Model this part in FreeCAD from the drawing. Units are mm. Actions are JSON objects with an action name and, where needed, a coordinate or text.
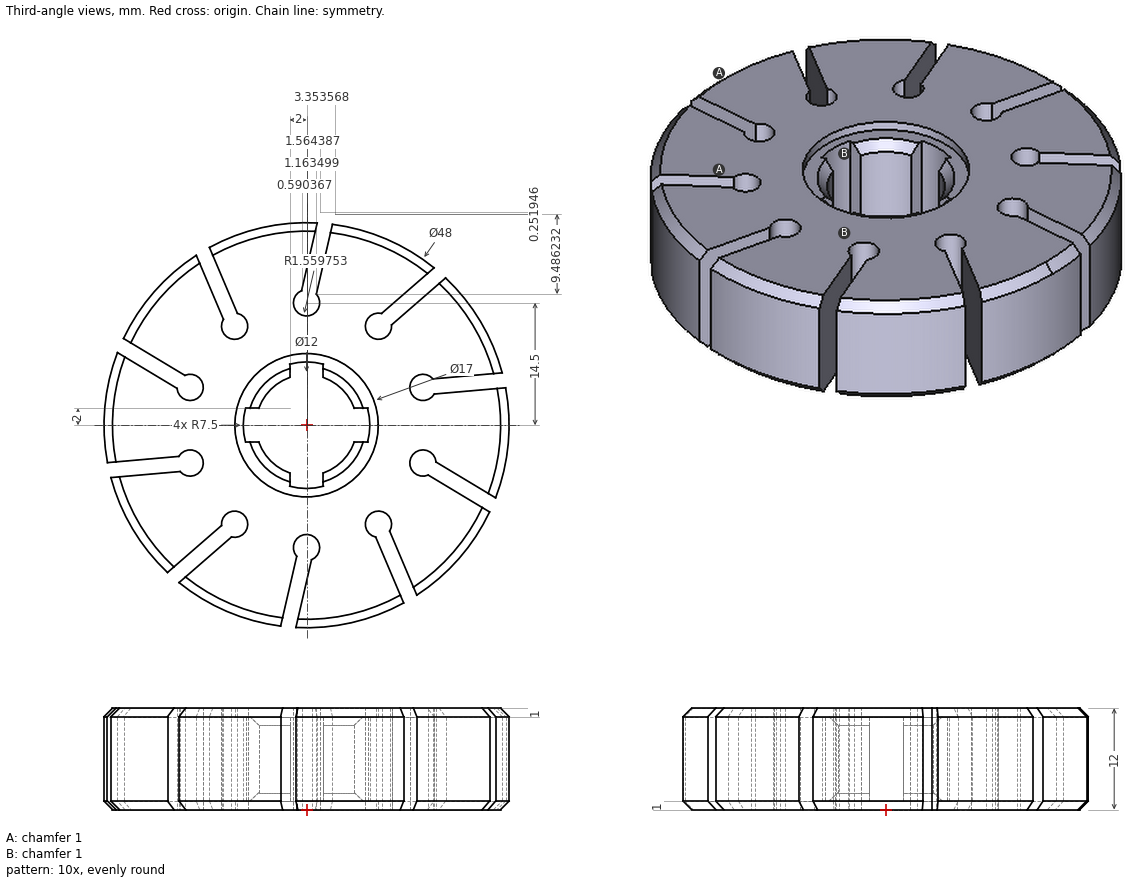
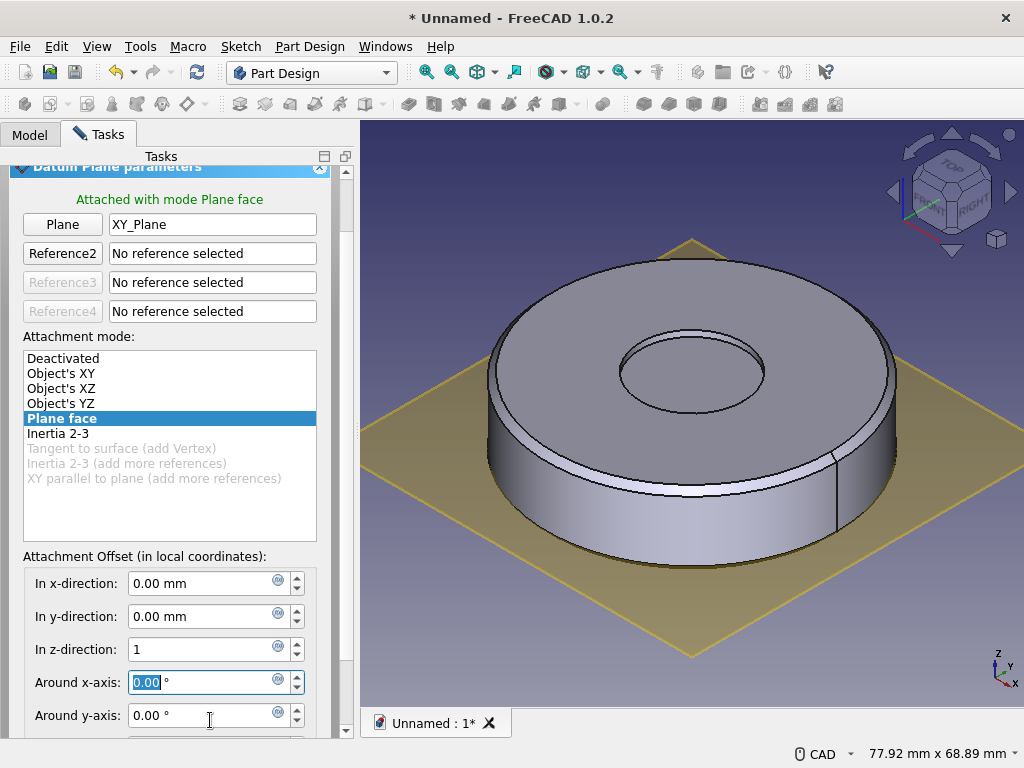
{"action": "scroll", "coordinate": [346, 452], "scroll_direction": "up", "scroll_amount": 2}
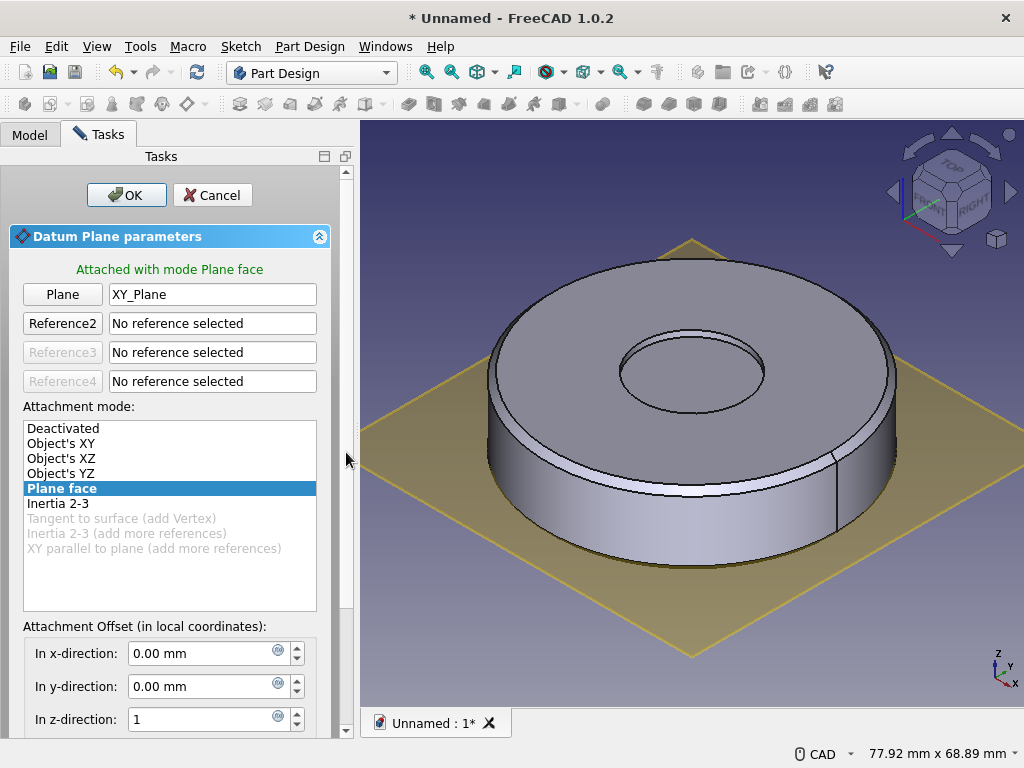
{"action": "left_click", "coordinate": [127, 195]}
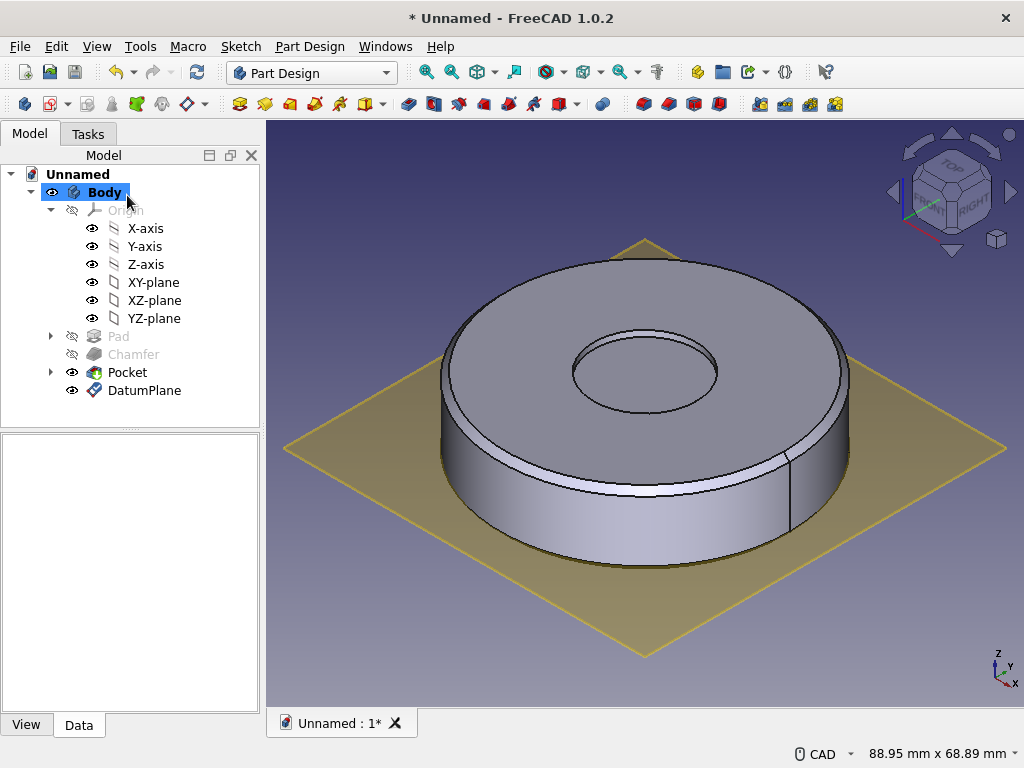
{"action": "left_click", "coordinate": [117, 390]}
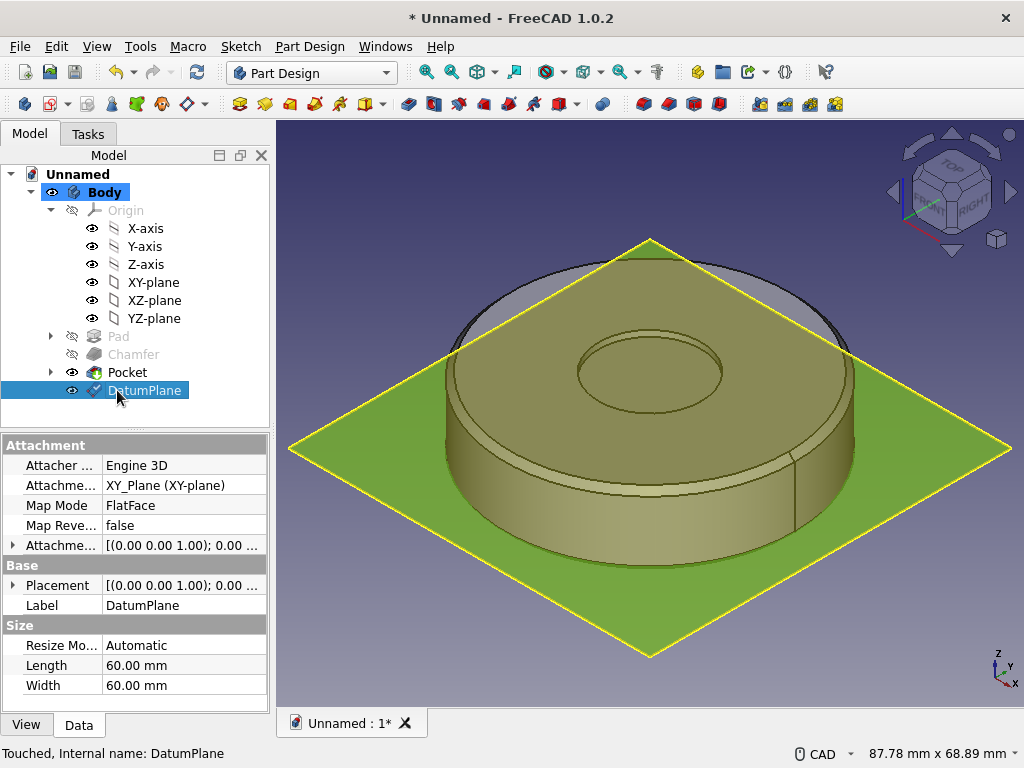
{"action": "left_click", "coordinate": [50, 104]}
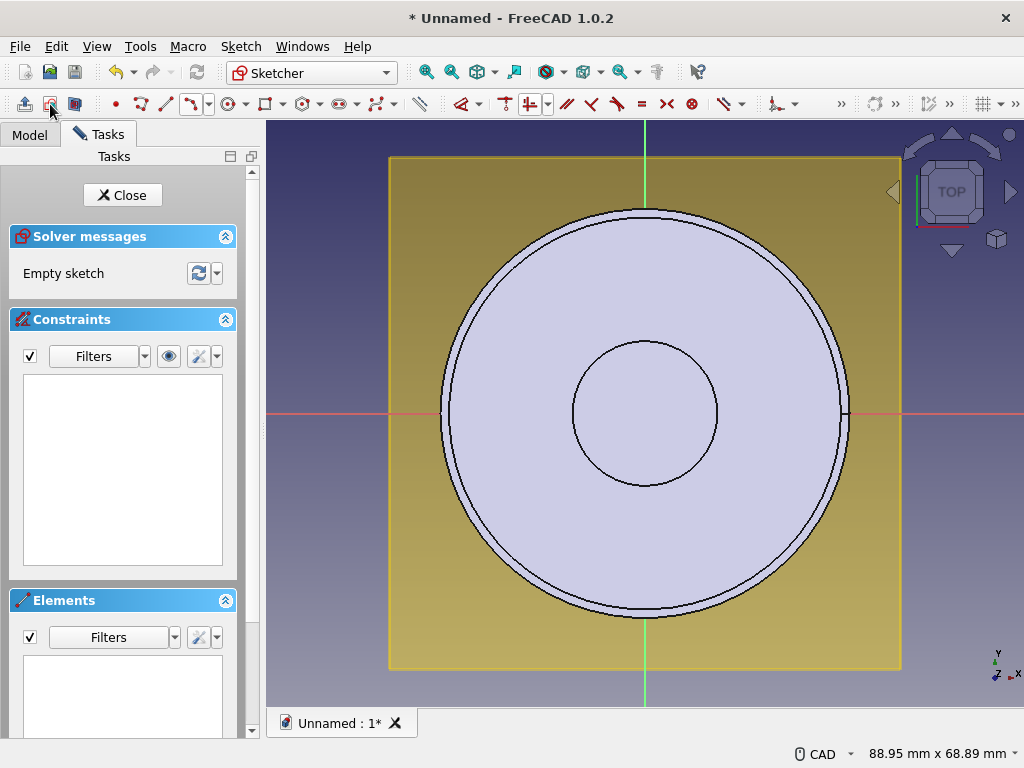
{"action": "left_click", "coordinate": [75, 104]}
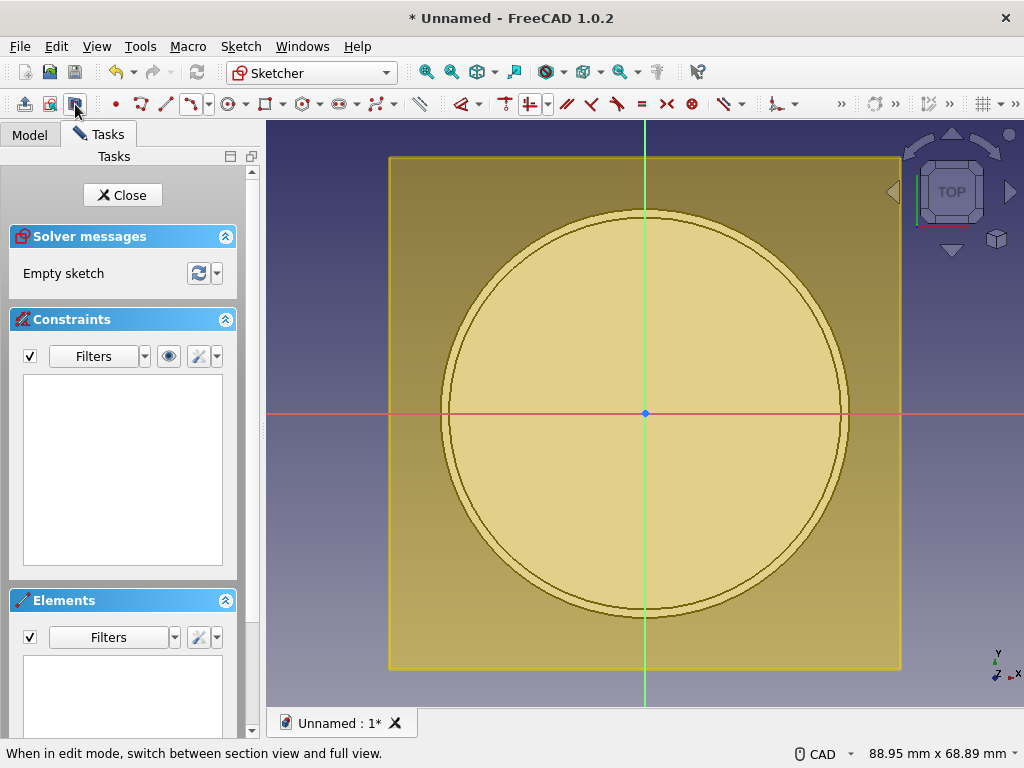
{"action": "scroll", "coordinate": [685, 413], "scroll_direction": "up", "scroll_amount": 5}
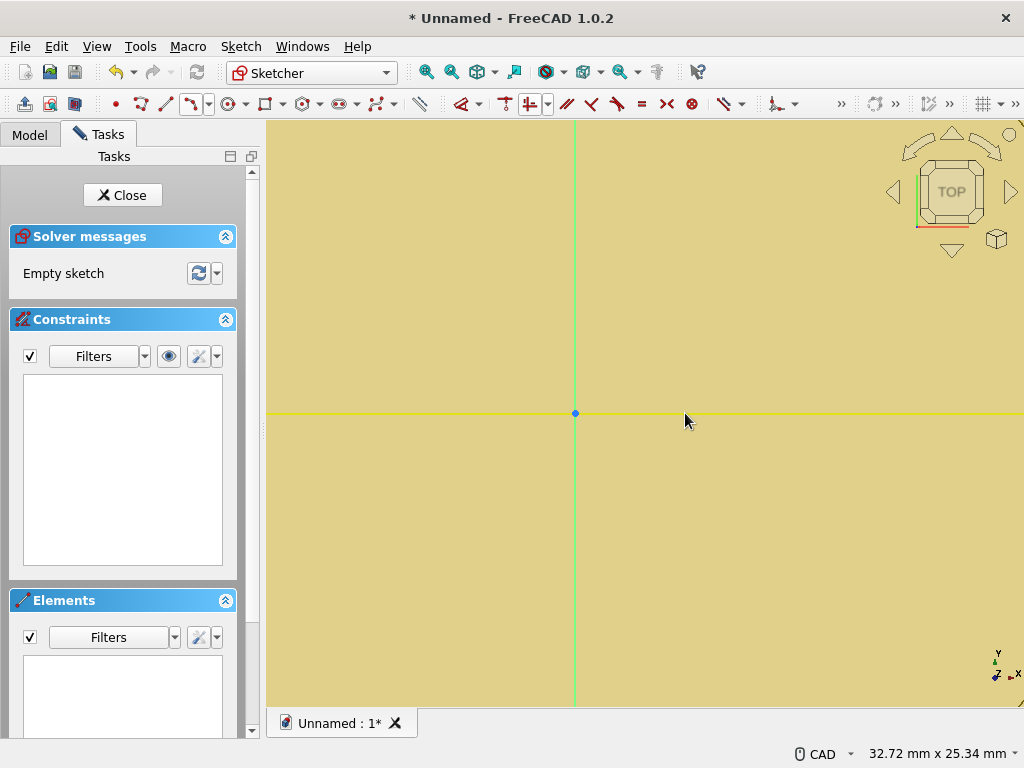
{"action": "left_click", "coordinate": [228, 104]}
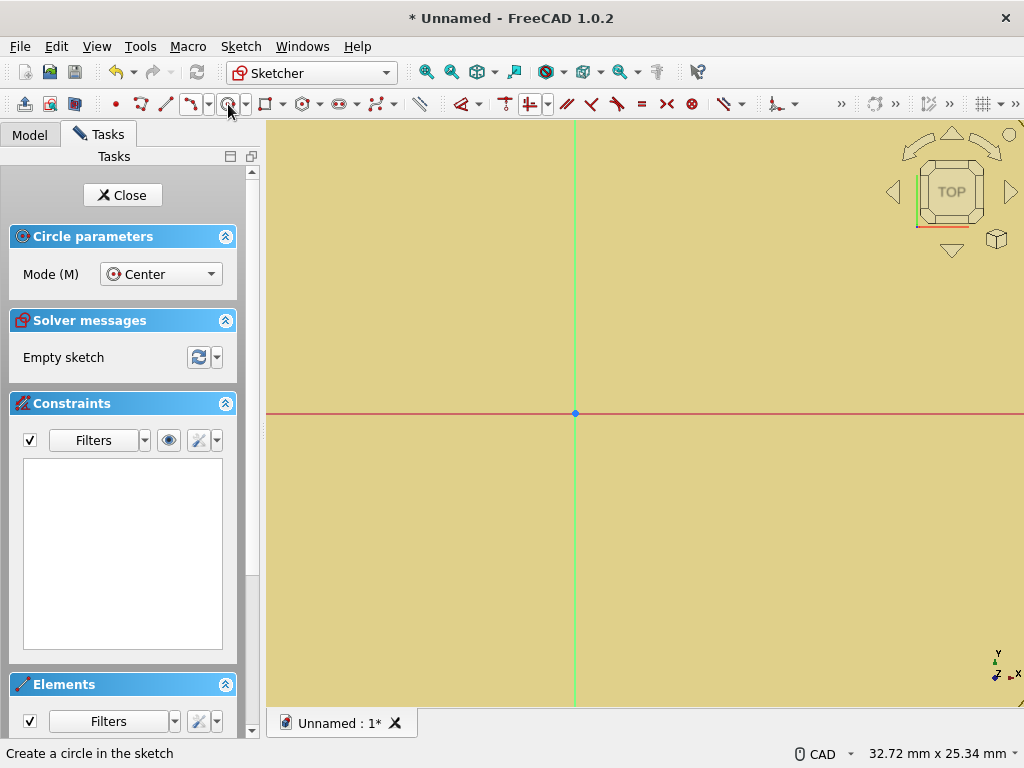
{"action": "left_click", "coordinate": [575, 413]}
{"action": "mouse_move", "coordinate": [715, 274]}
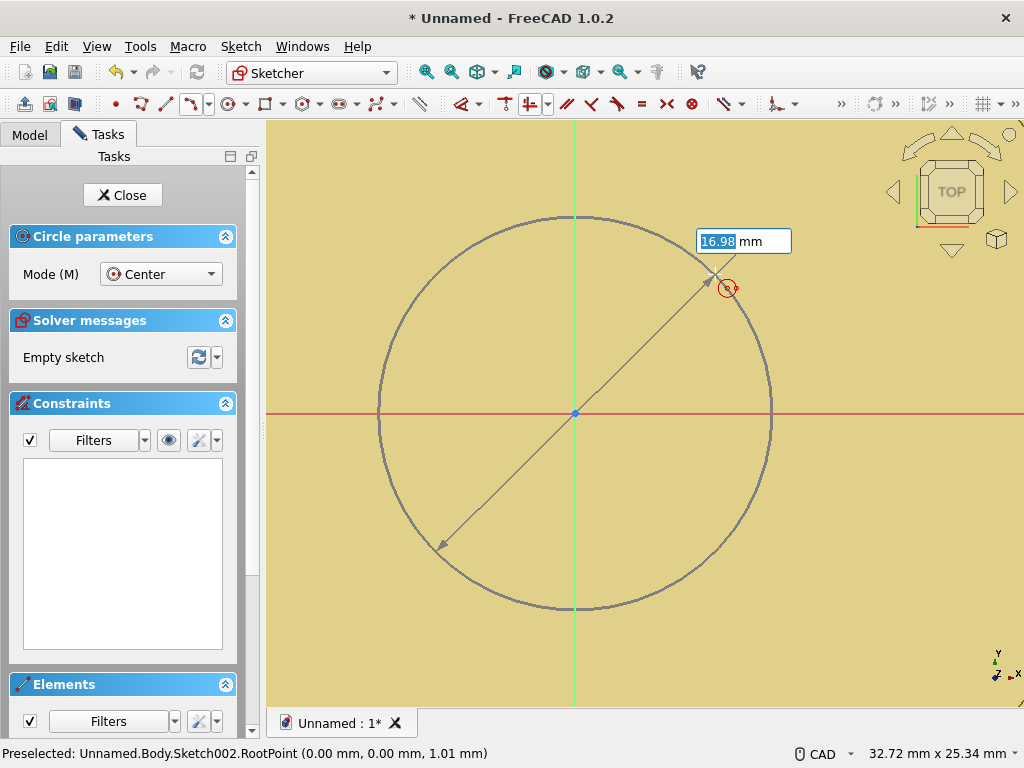
{"action": "type", "text": "17"}
{"action": "key", "text": "Return"}
{"action": "key", "text": "Escape"}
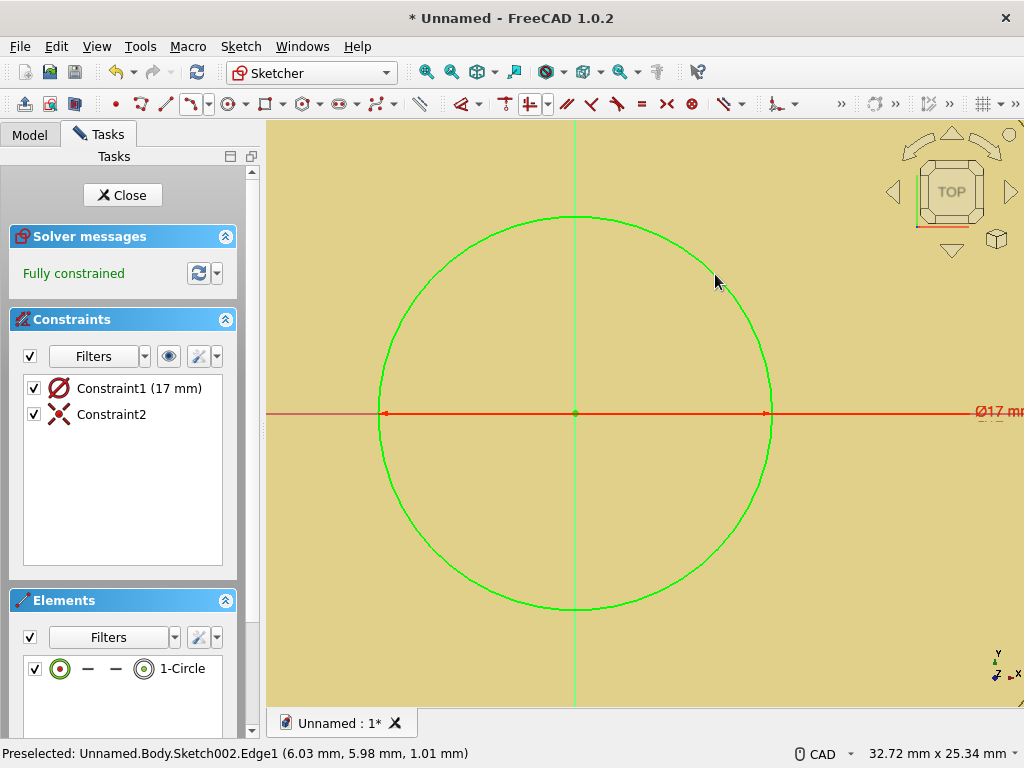
{"action": "left_click", "coordinate": [123, 195]}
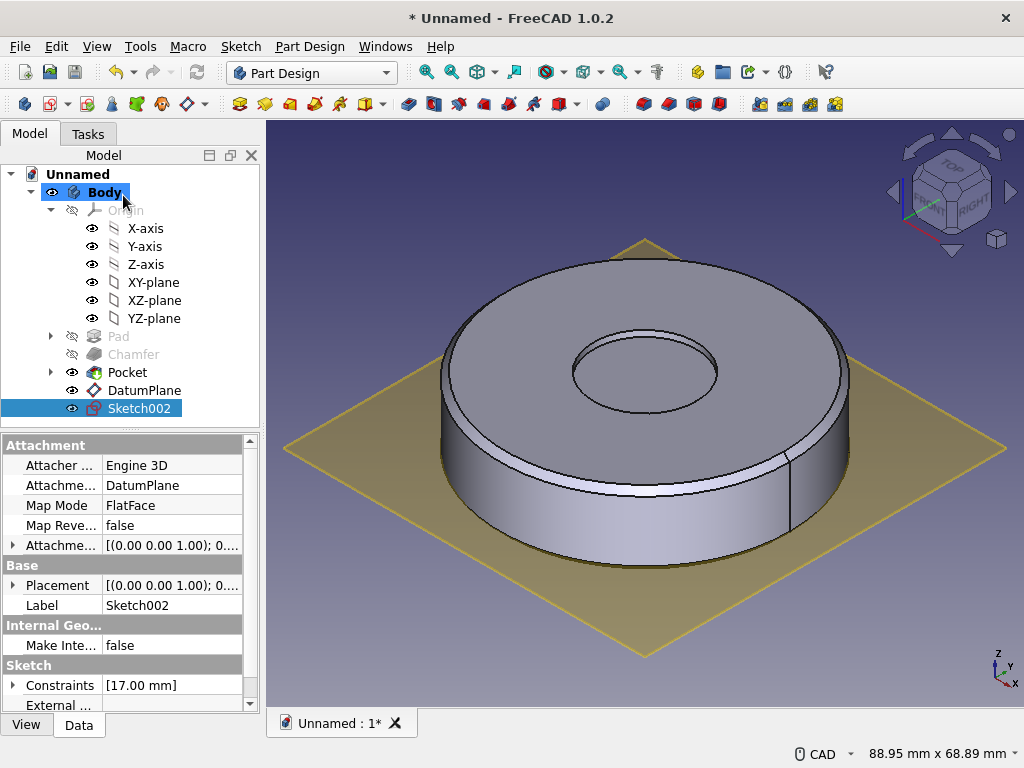
{"action": "left_click", "coordinate": [409, 104]}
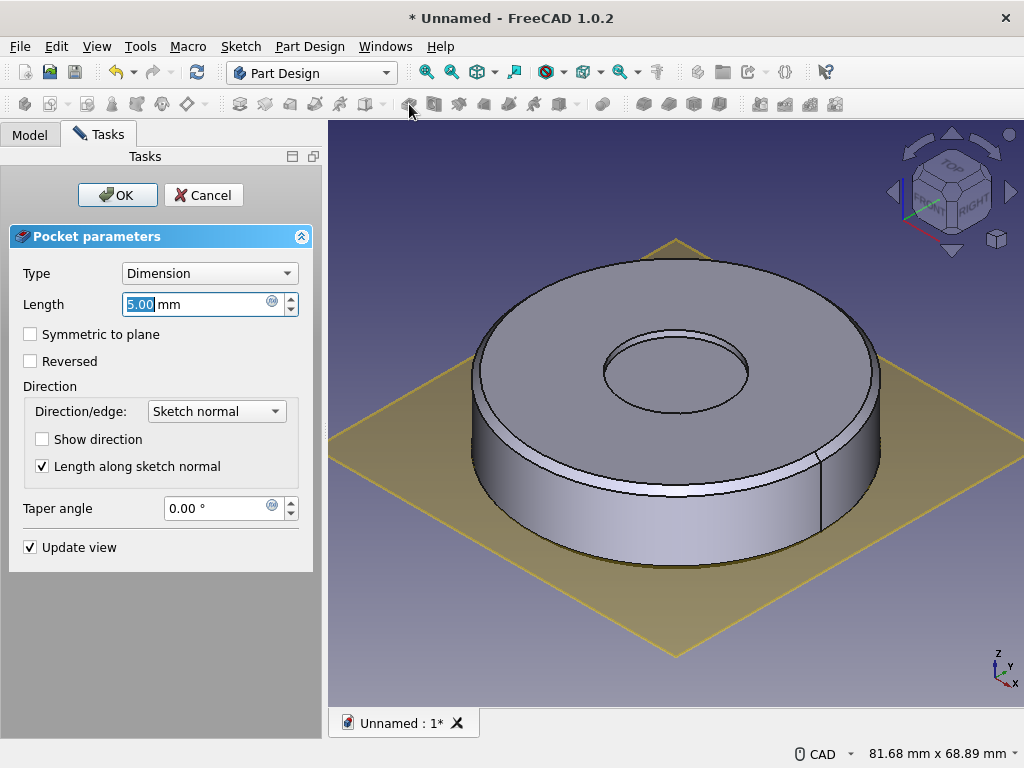
{"action": "type", "text": "1"}
{"action": "key", "text": "Tab"}